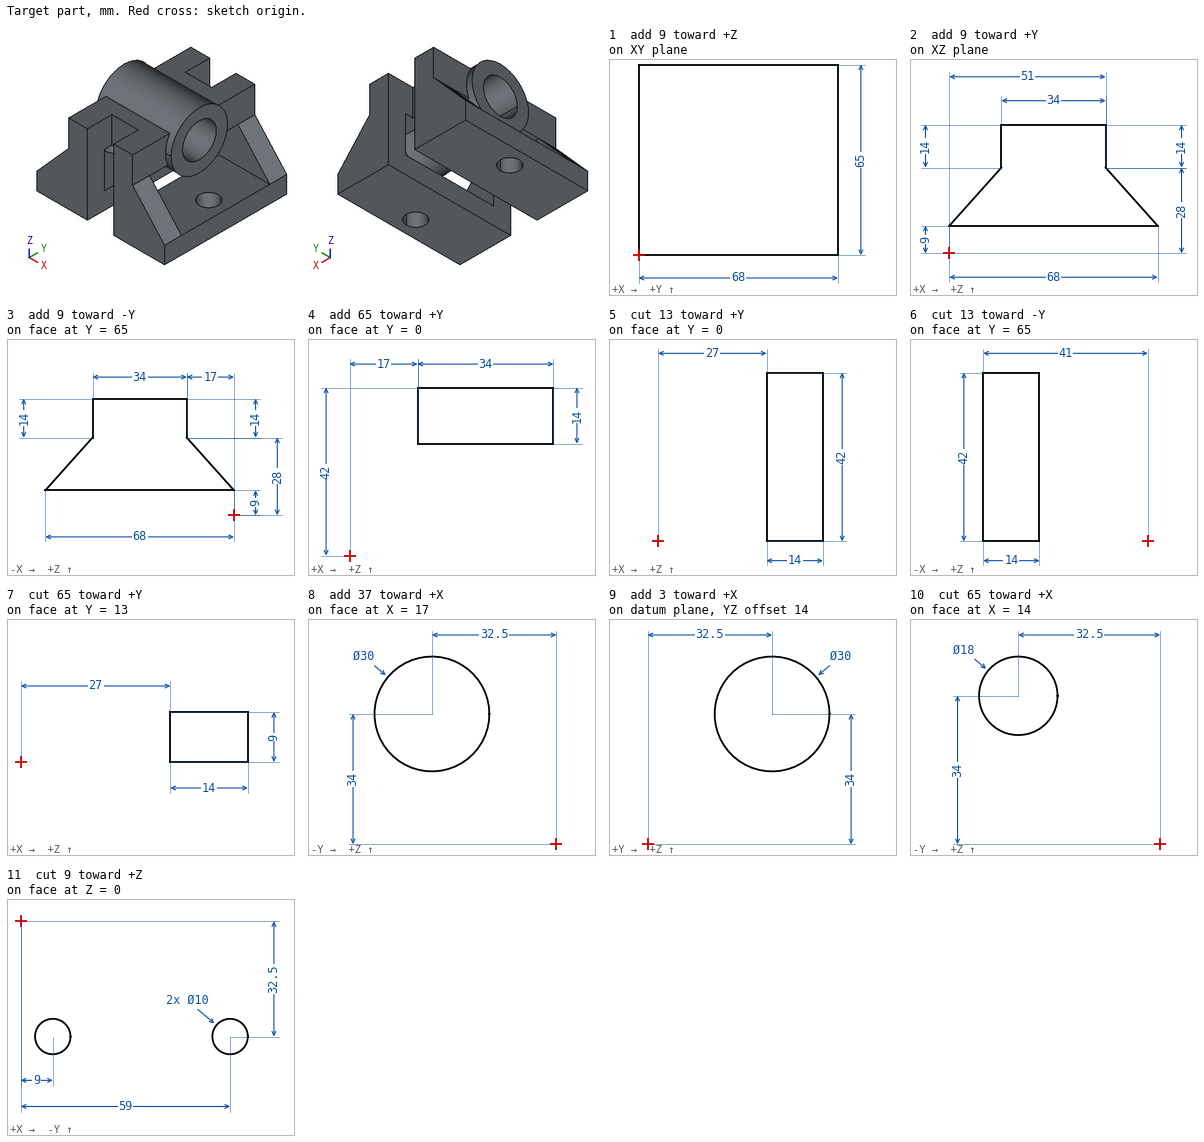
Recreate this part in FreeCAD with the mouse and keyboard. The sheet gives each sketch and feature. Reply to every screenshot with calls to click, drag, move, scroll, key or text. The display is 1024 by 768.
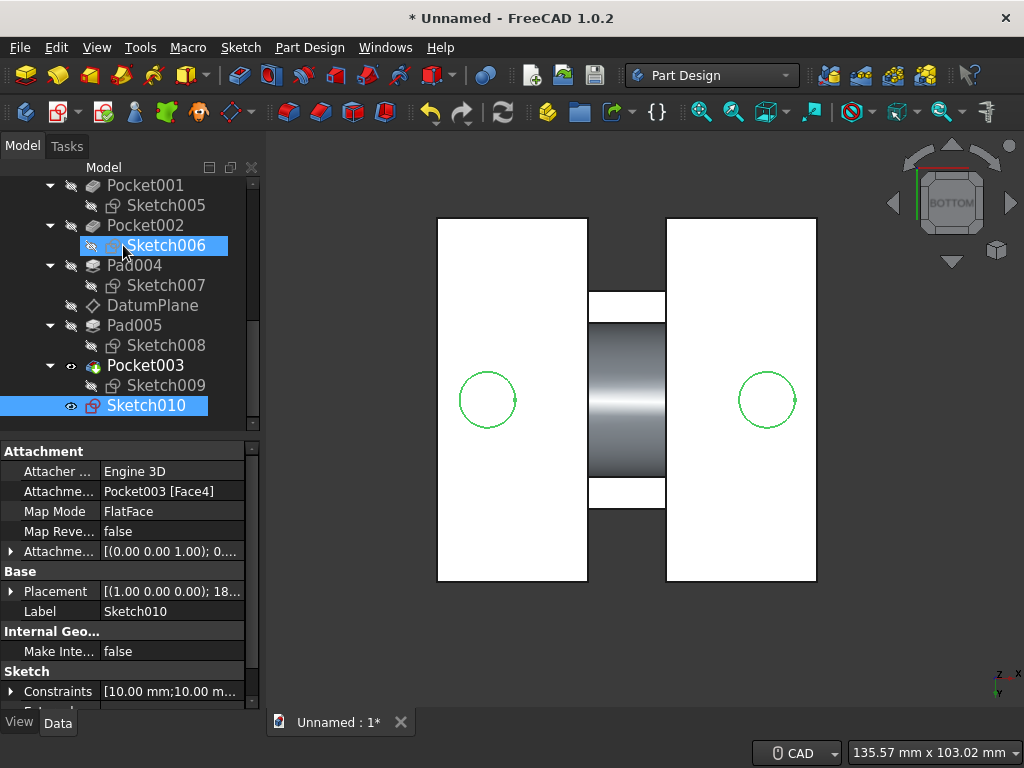
click(240, 76)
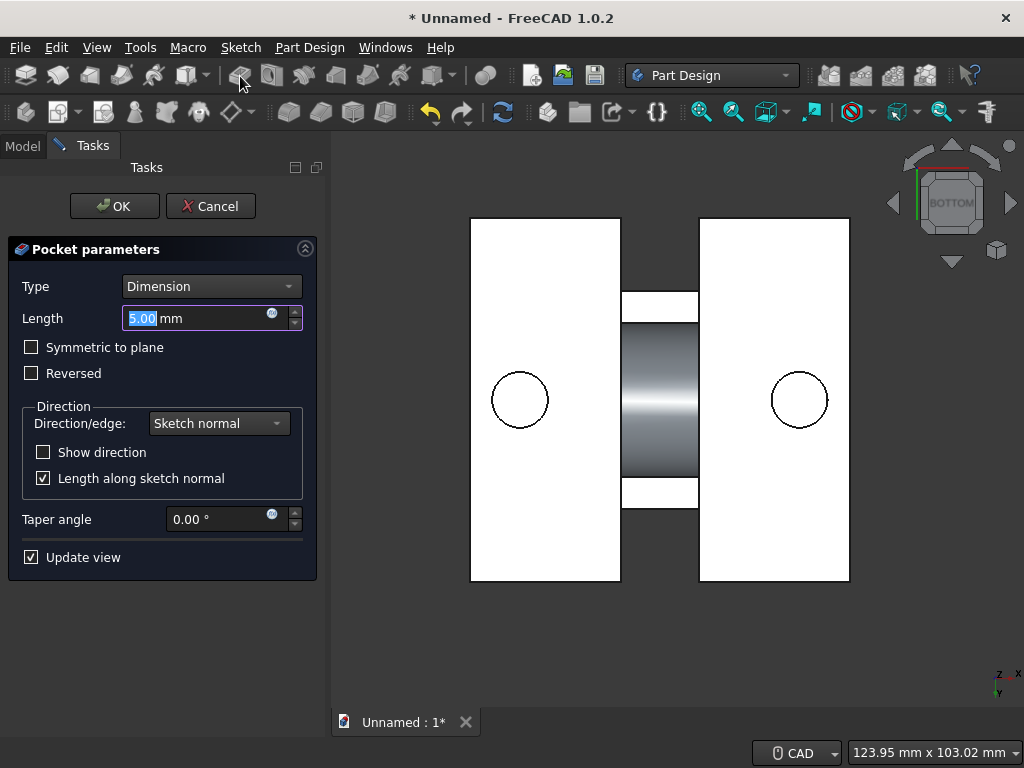
text(9)
key(Tab)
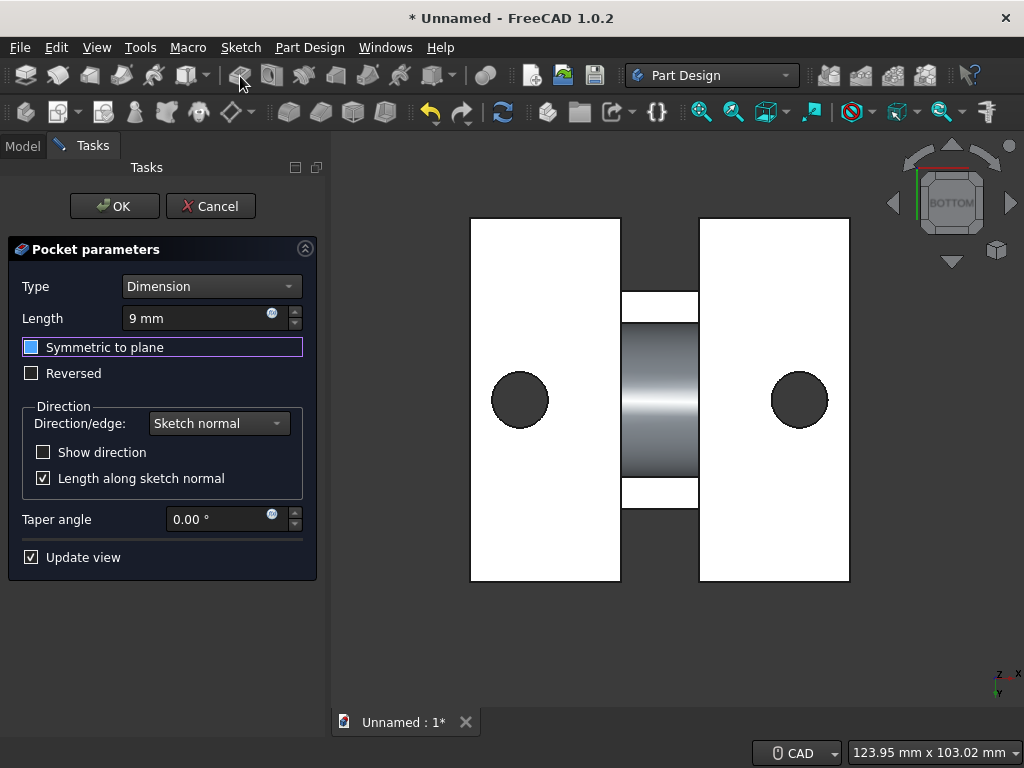
click(115, 206)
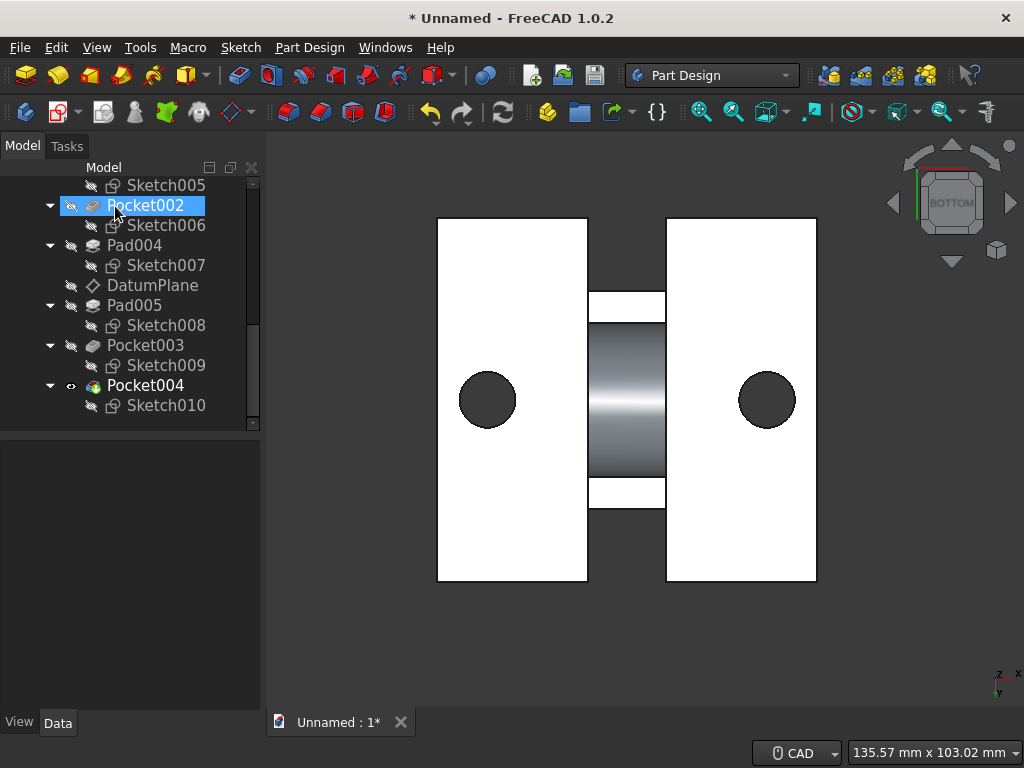
key(0)